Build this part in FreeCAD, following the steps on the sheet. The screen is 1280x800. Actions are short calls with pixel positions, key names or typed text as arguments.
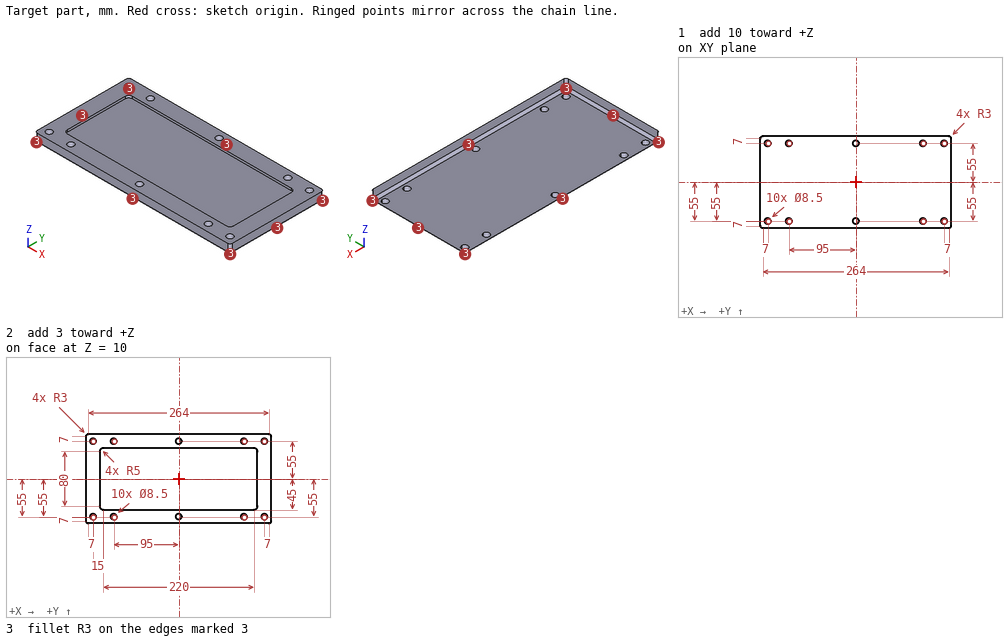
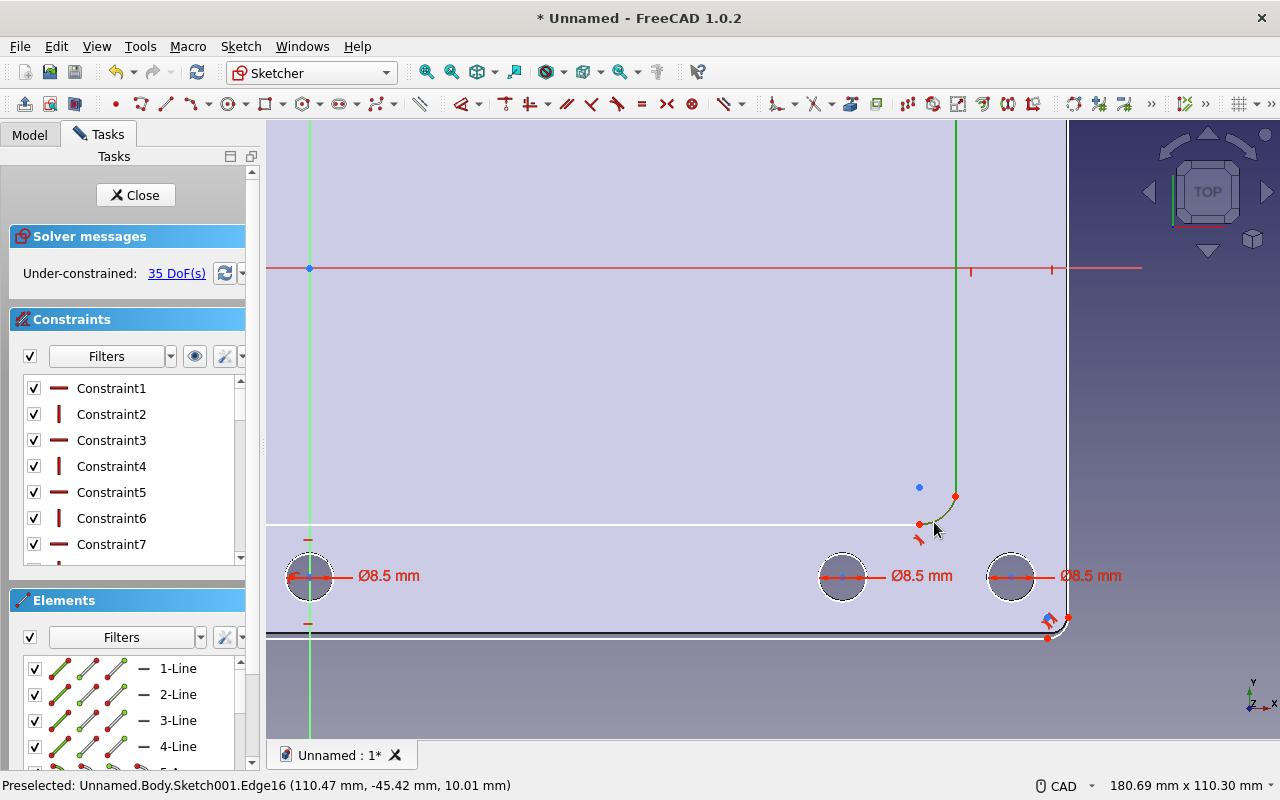
click(617, 104)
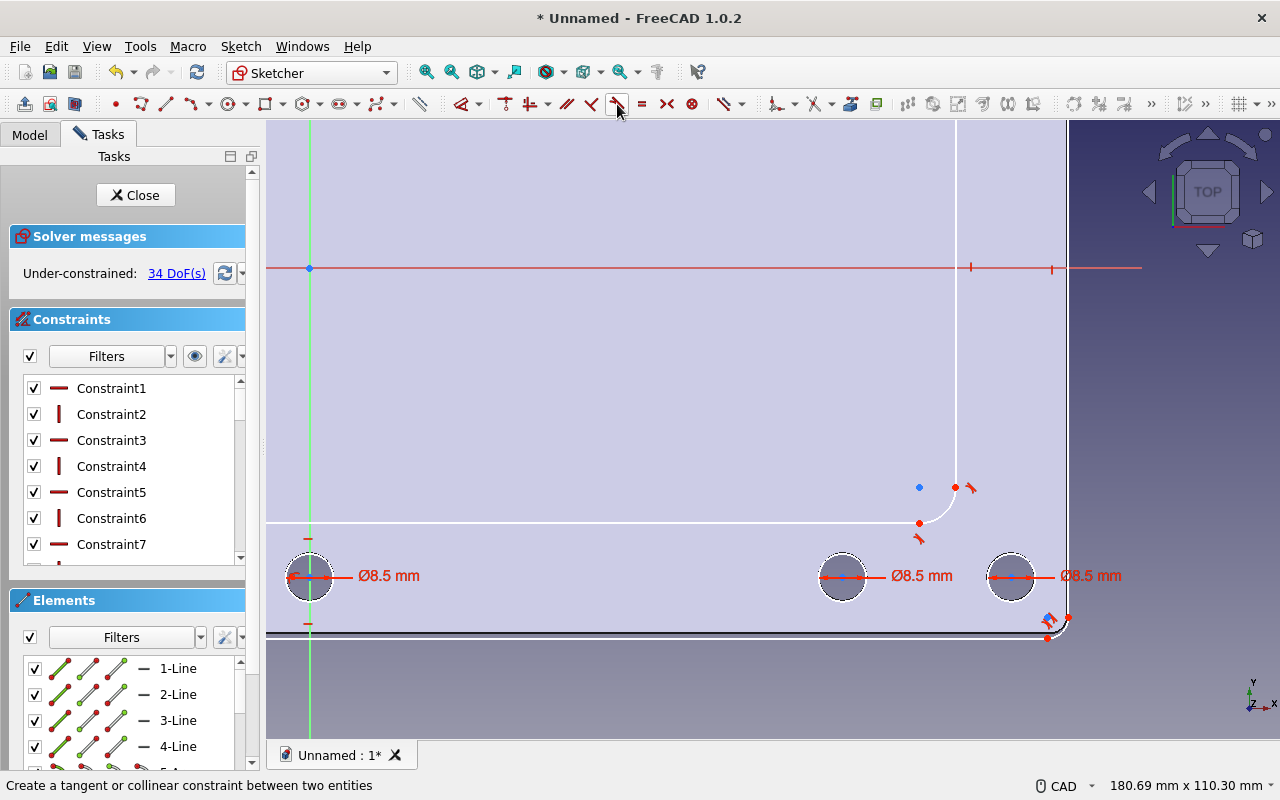
scroll(934, 523, down, 5)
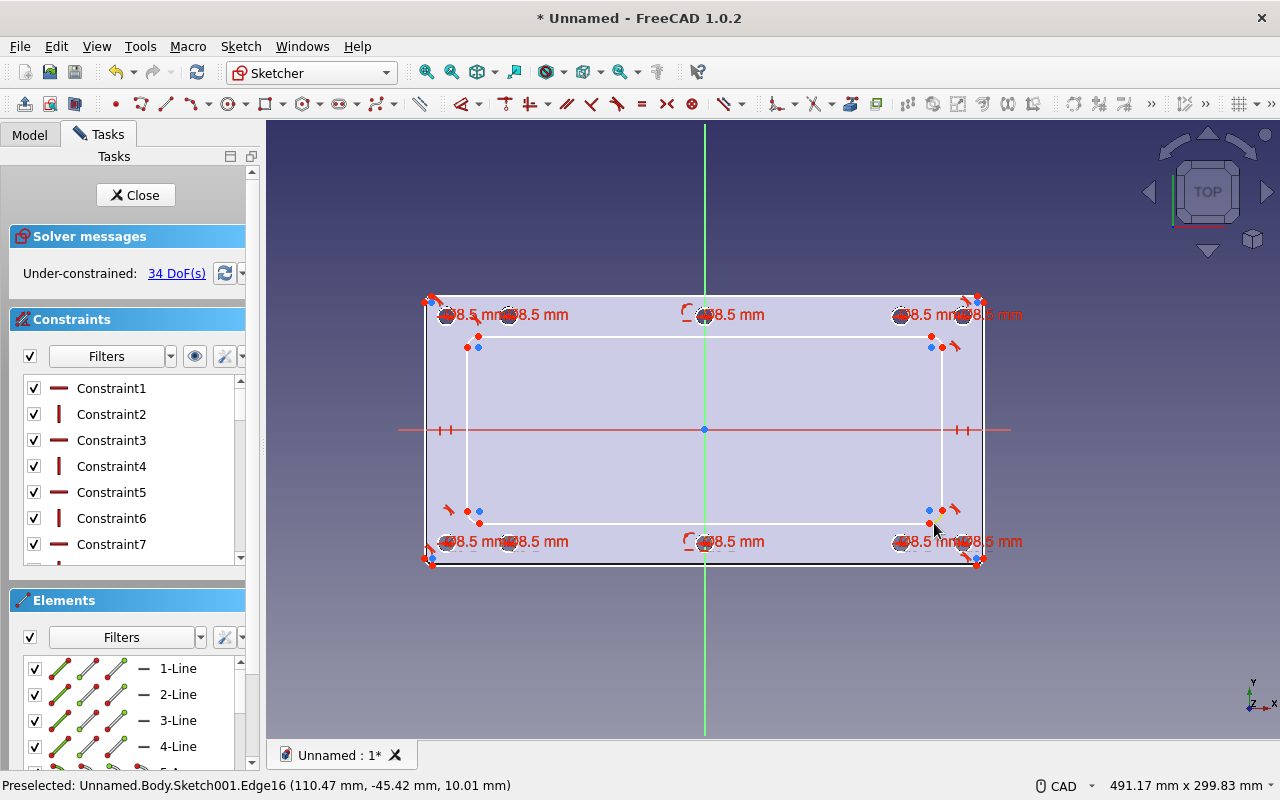
scroll(427, 298, up, 6)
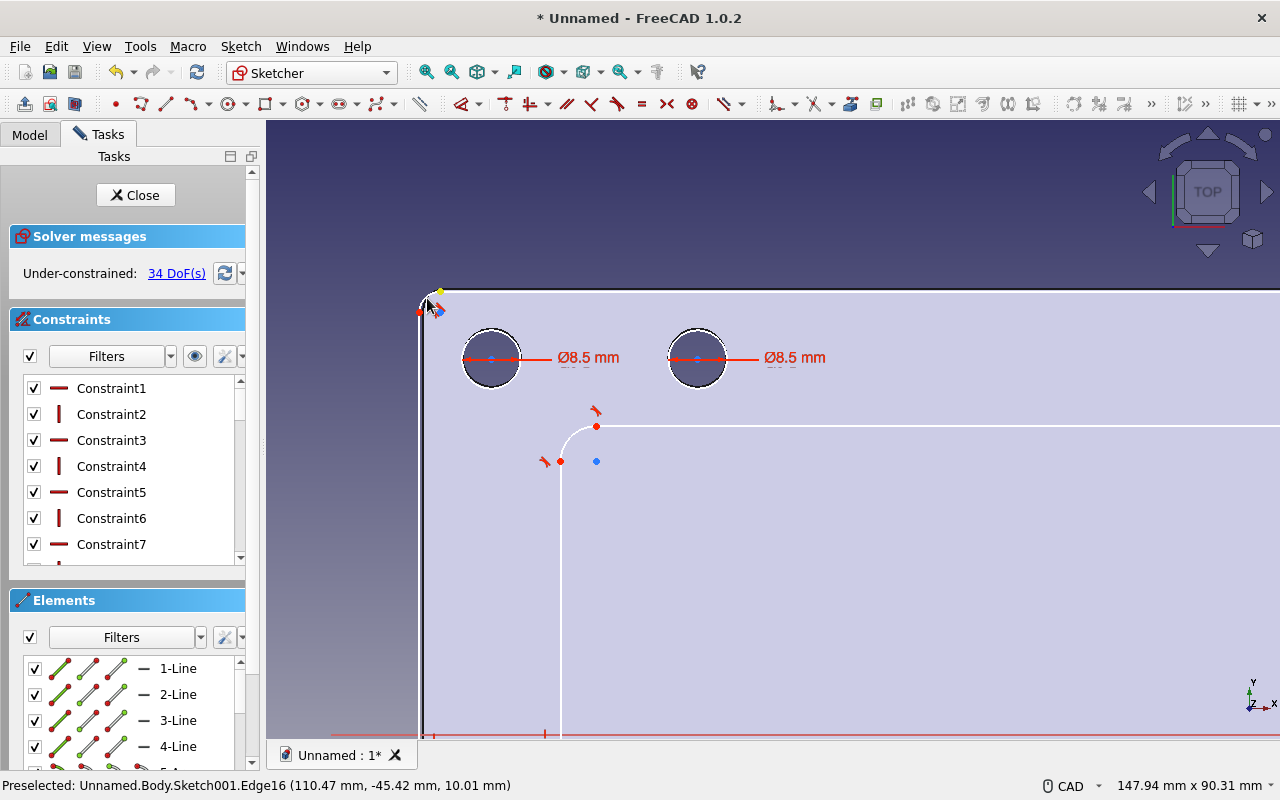
click(425, 298)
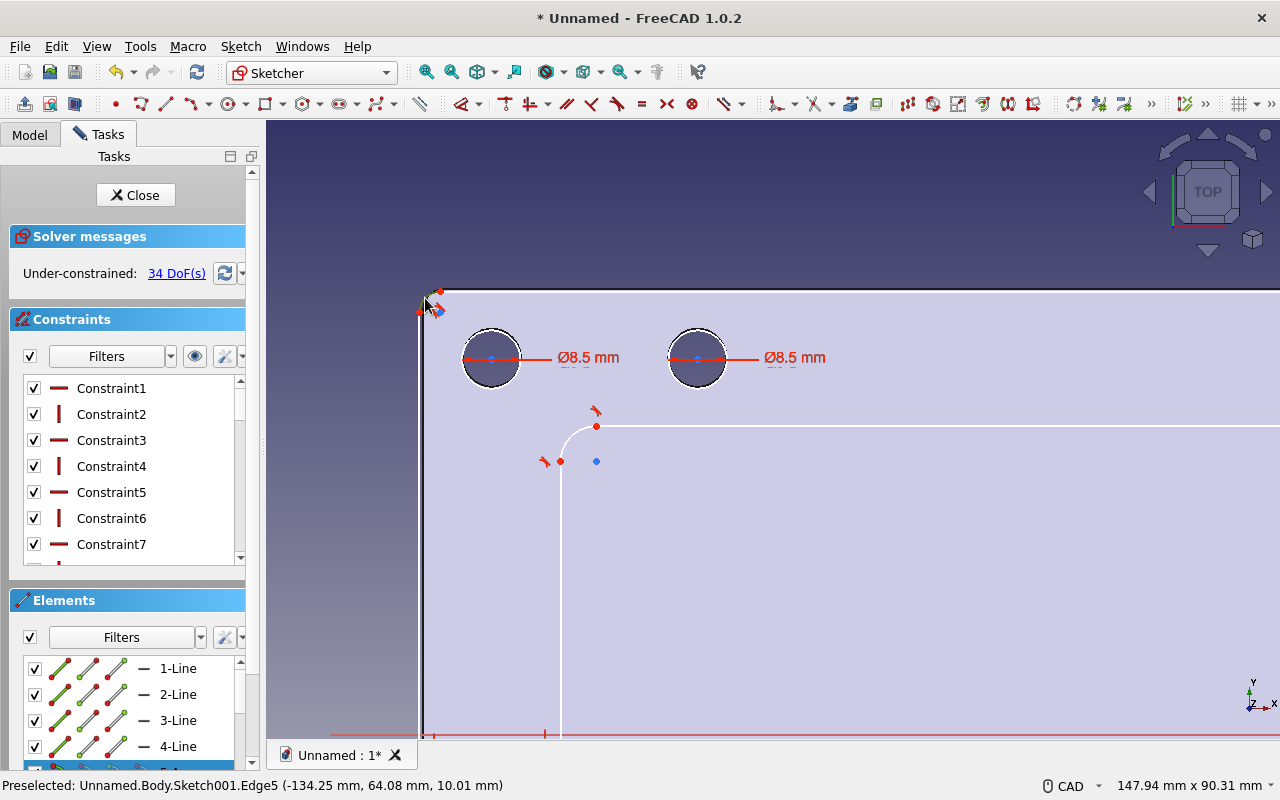
scroll(427, 298, down, 6)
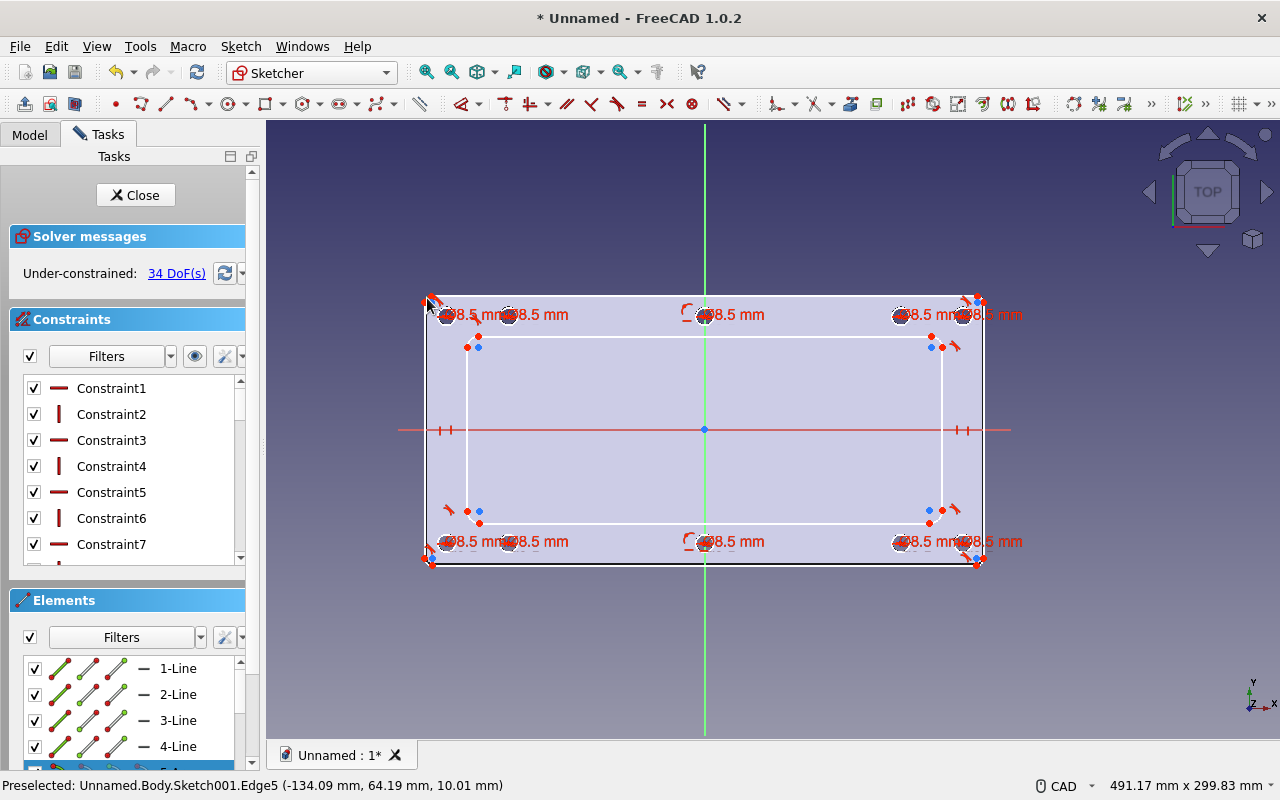
scroll(426, 562, up, 7)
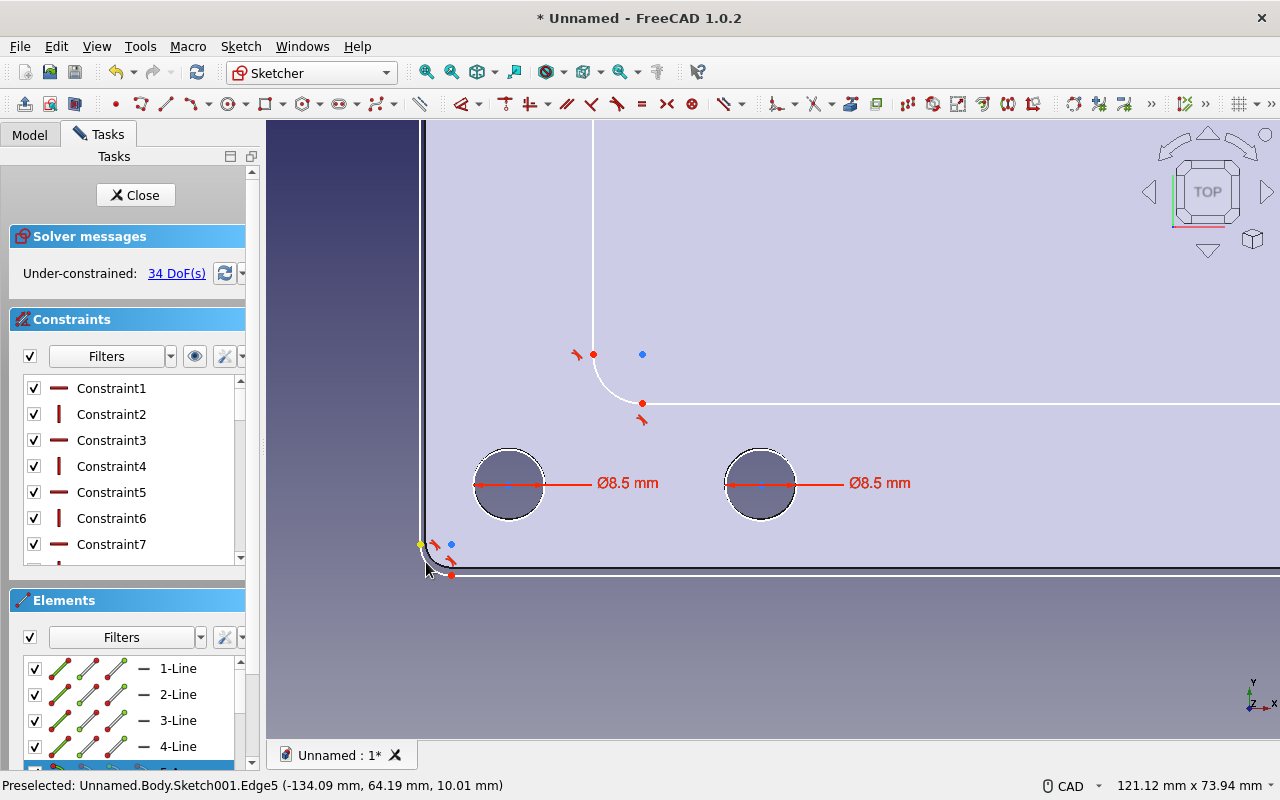
click(424, 559)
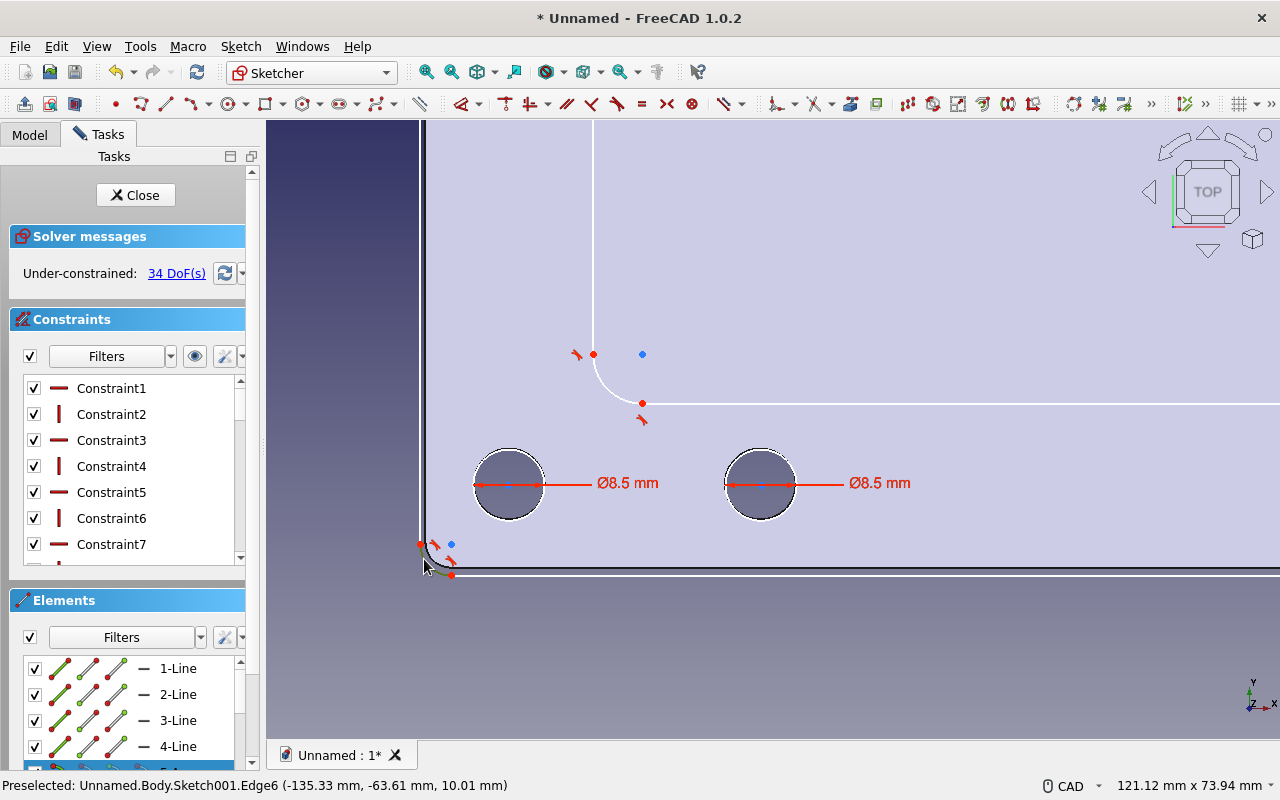
scroll(426, 562, down, 7)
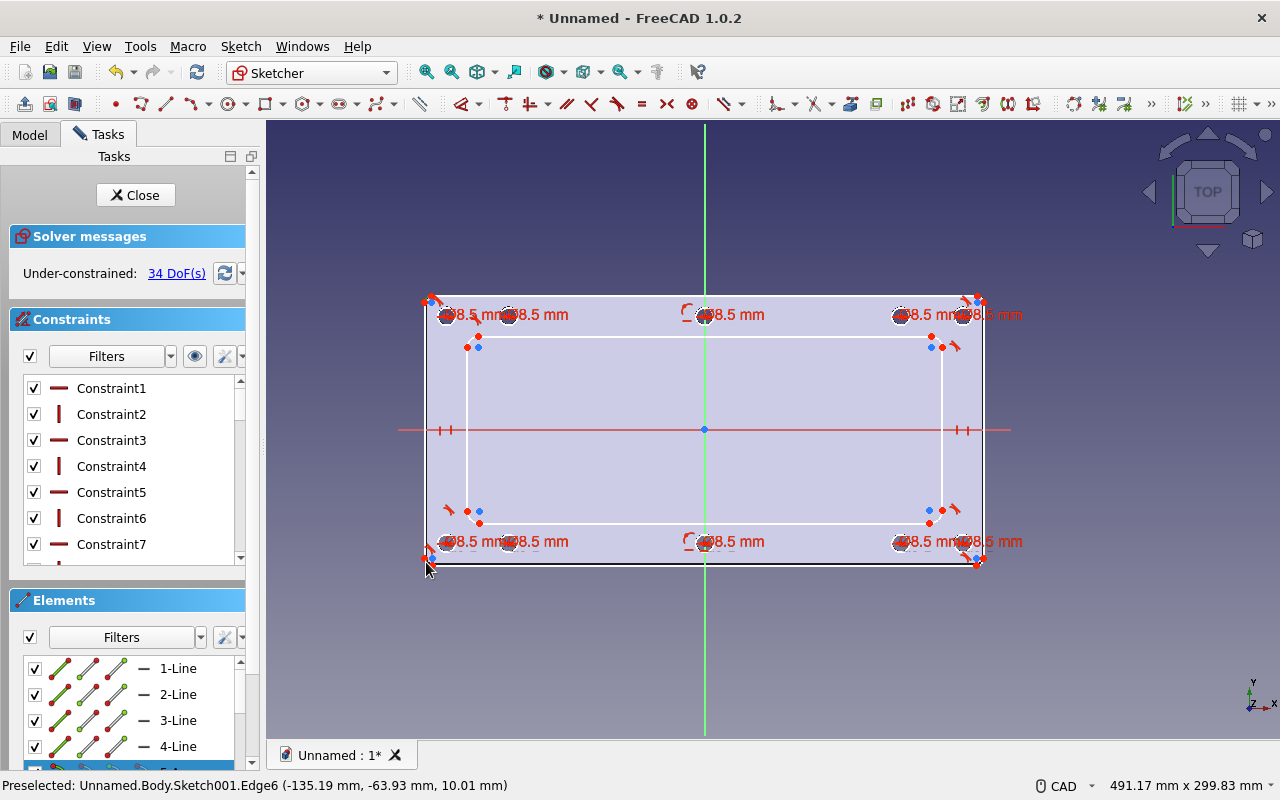
scroll(980, 565, up, 7)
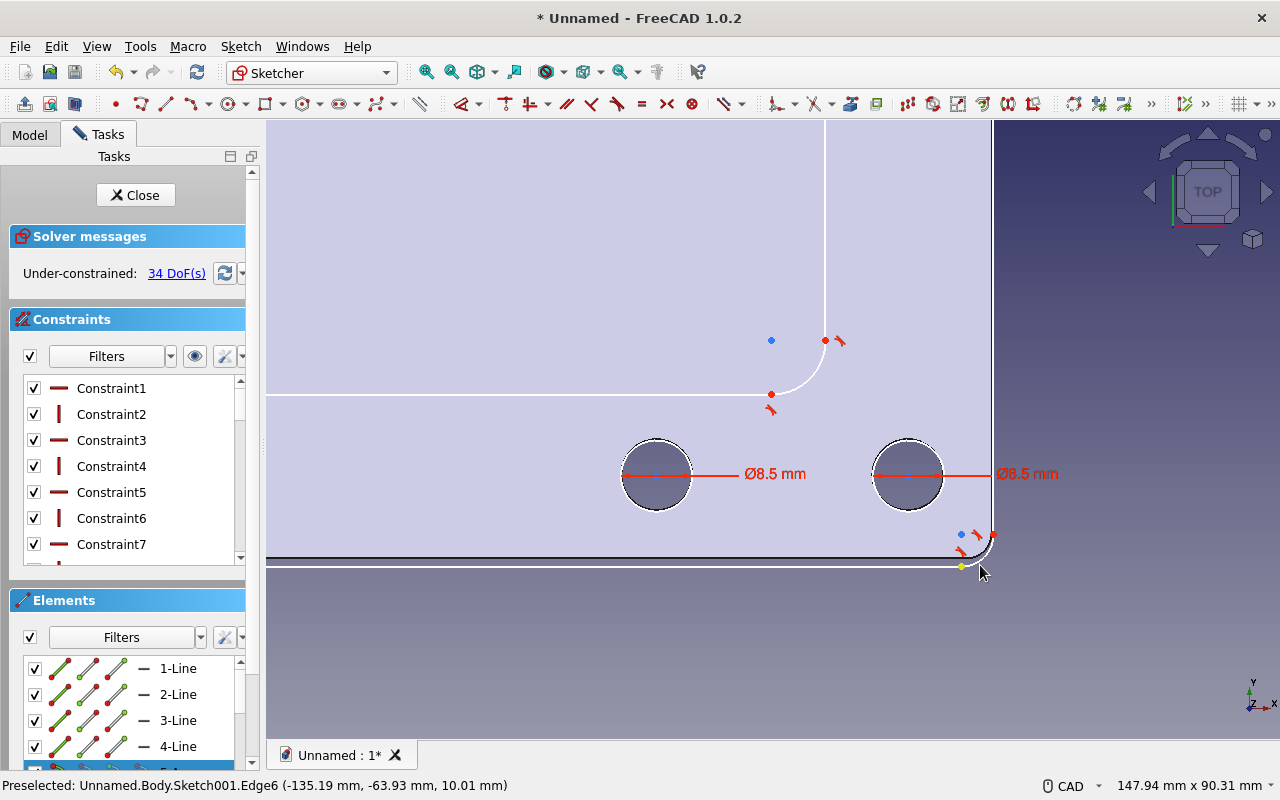
click(976, 563)